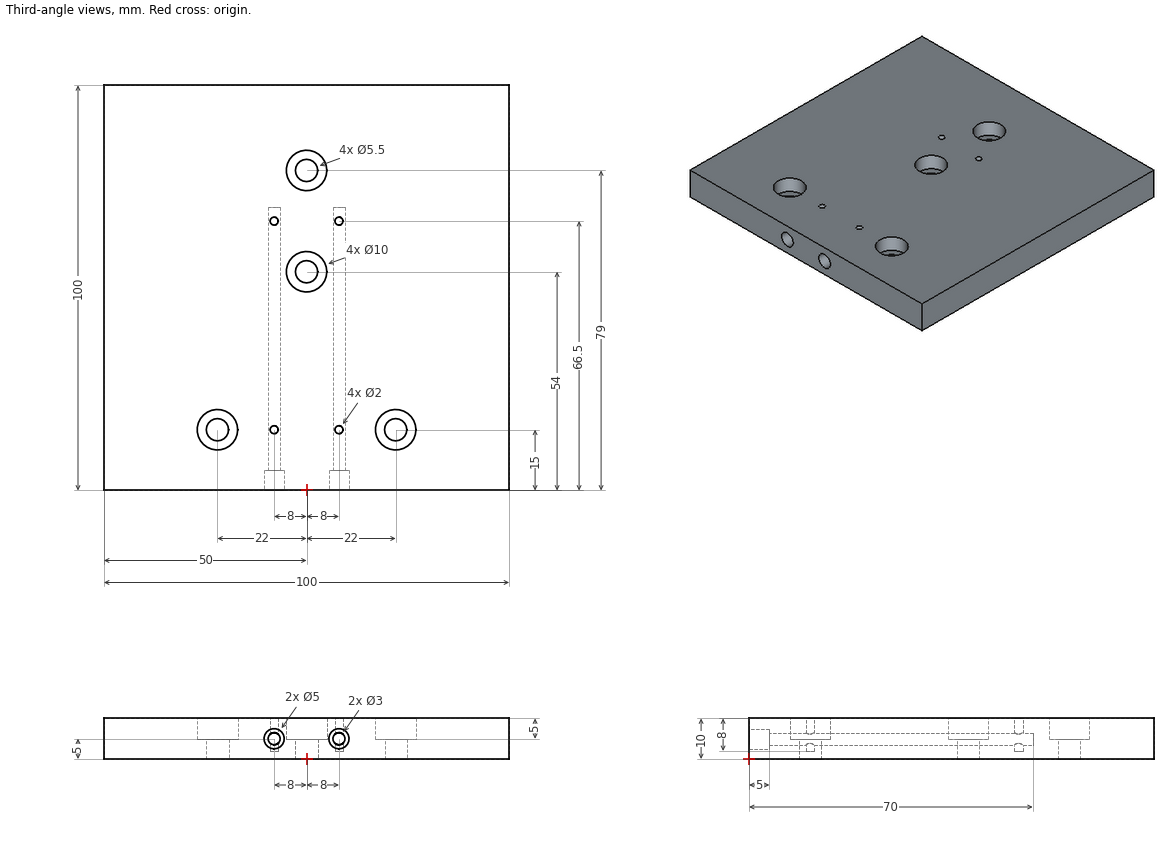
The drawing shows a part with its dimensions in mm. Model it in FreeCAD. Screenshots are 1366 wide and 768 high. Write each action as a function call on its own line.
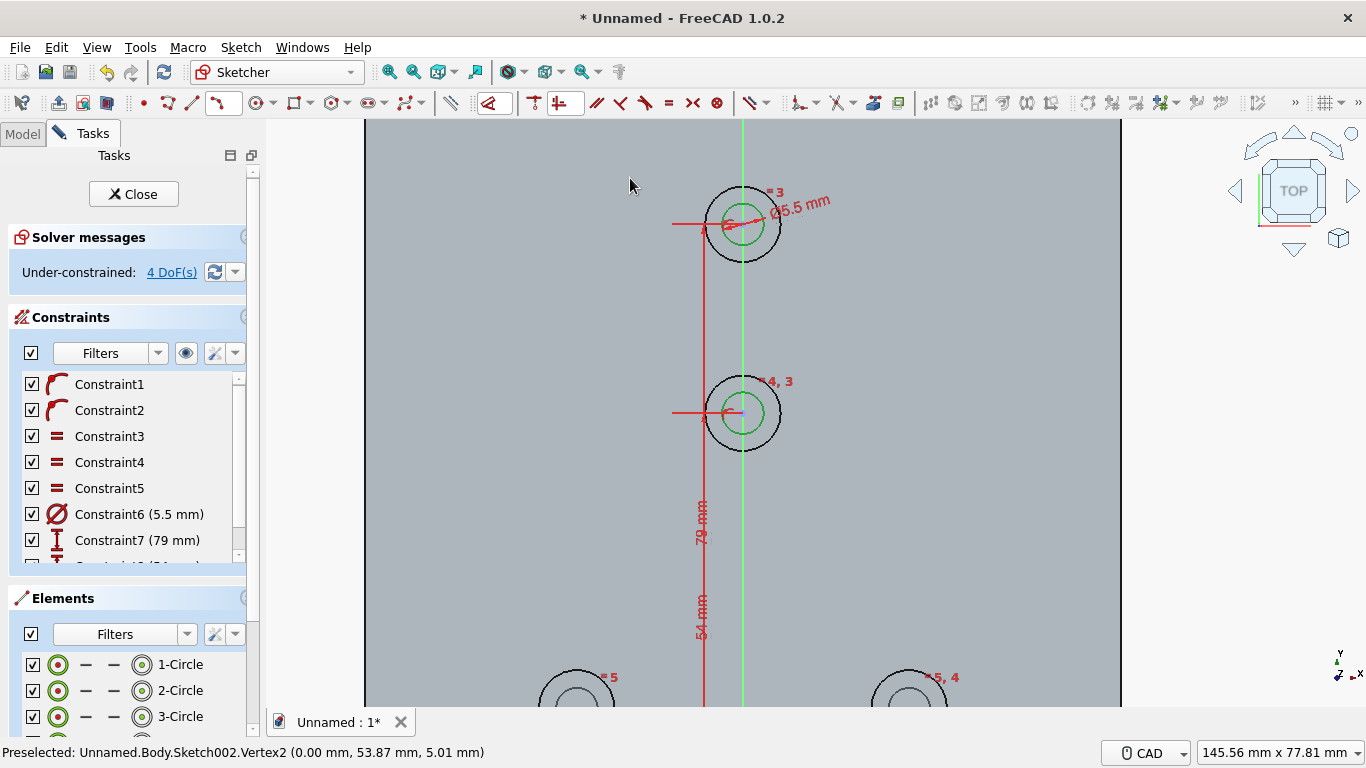
scroll(757, 211, down, 2)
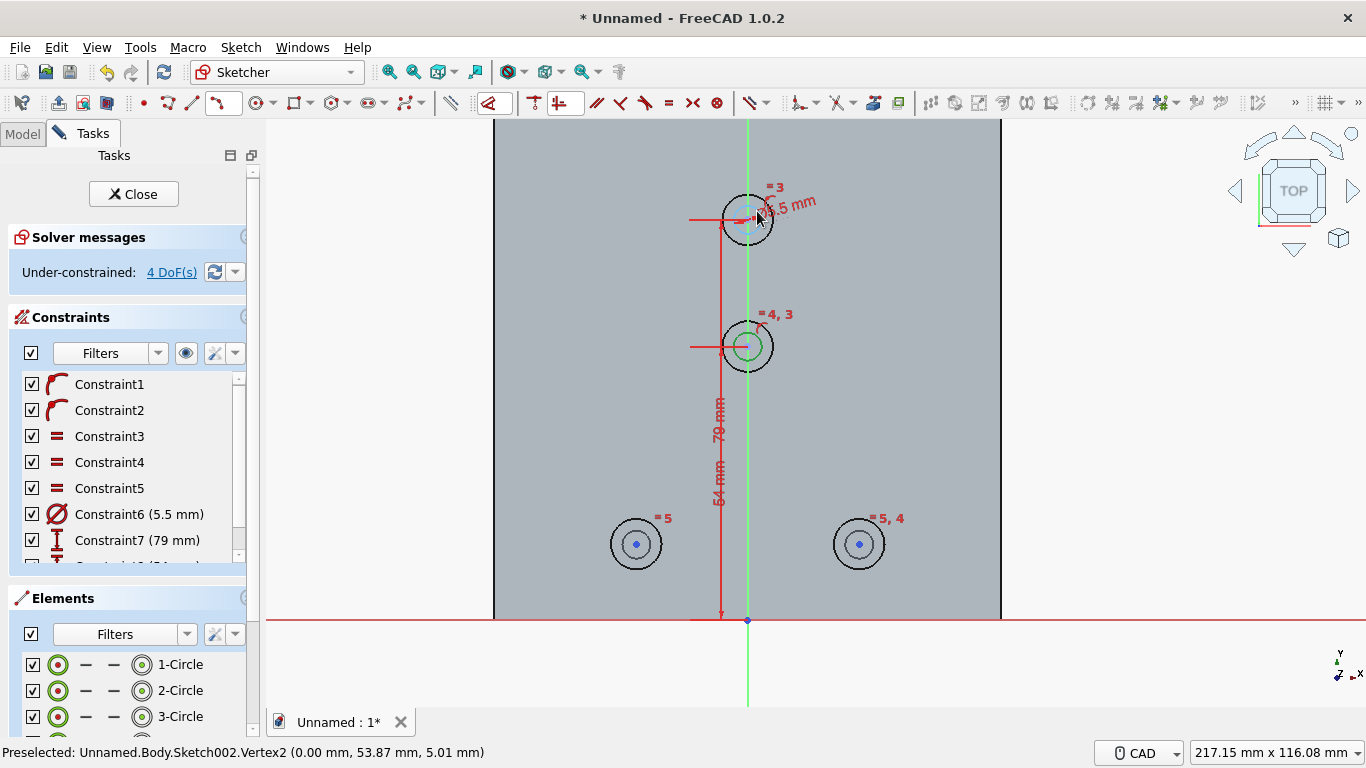
click(859, 545)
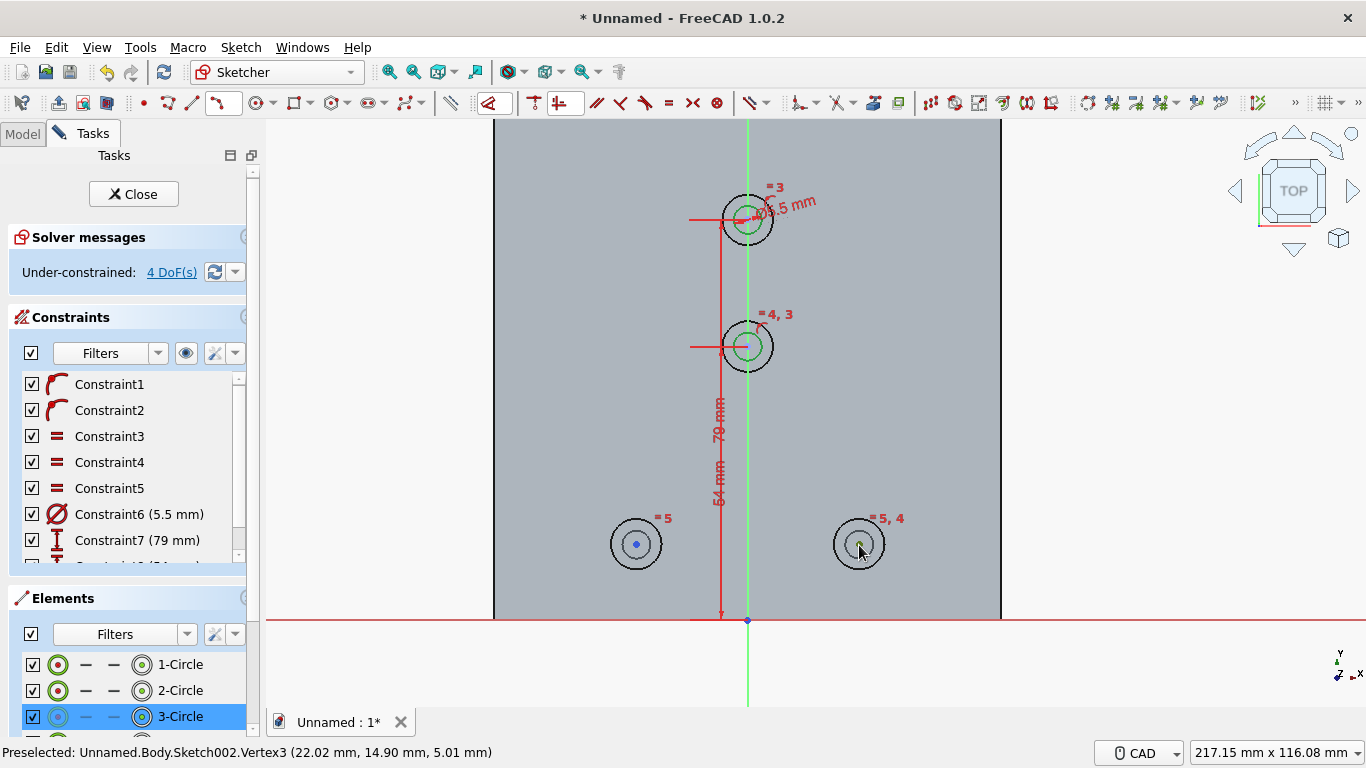
click(506, 104)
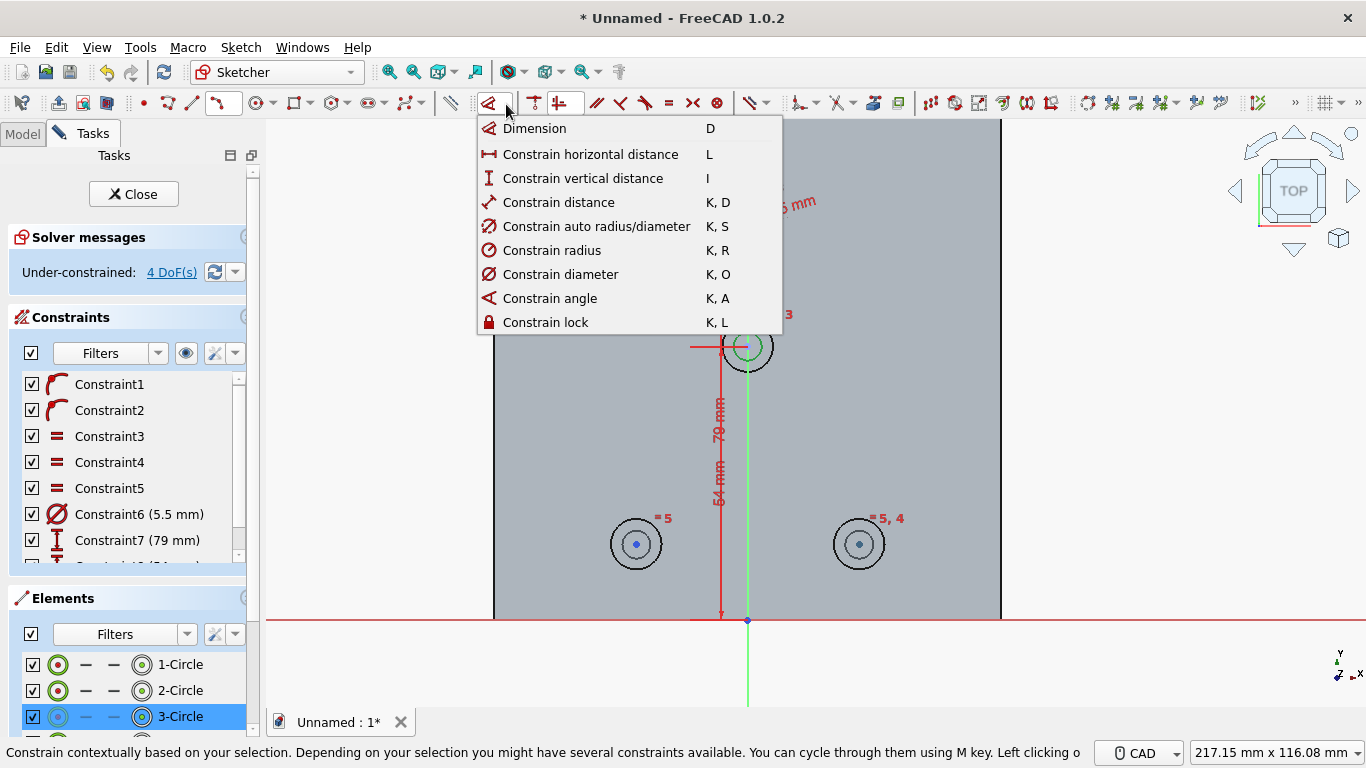
click(630, 154)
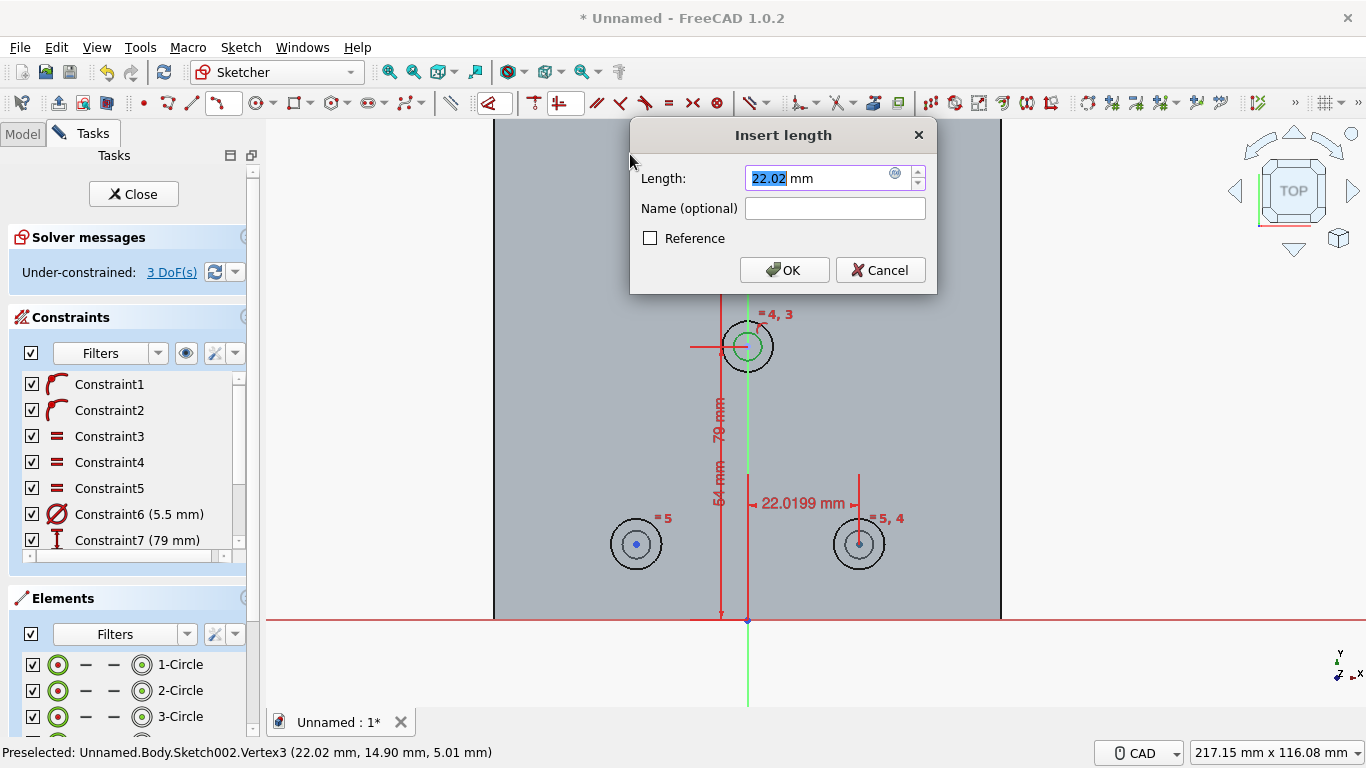
text(22)
key(Return)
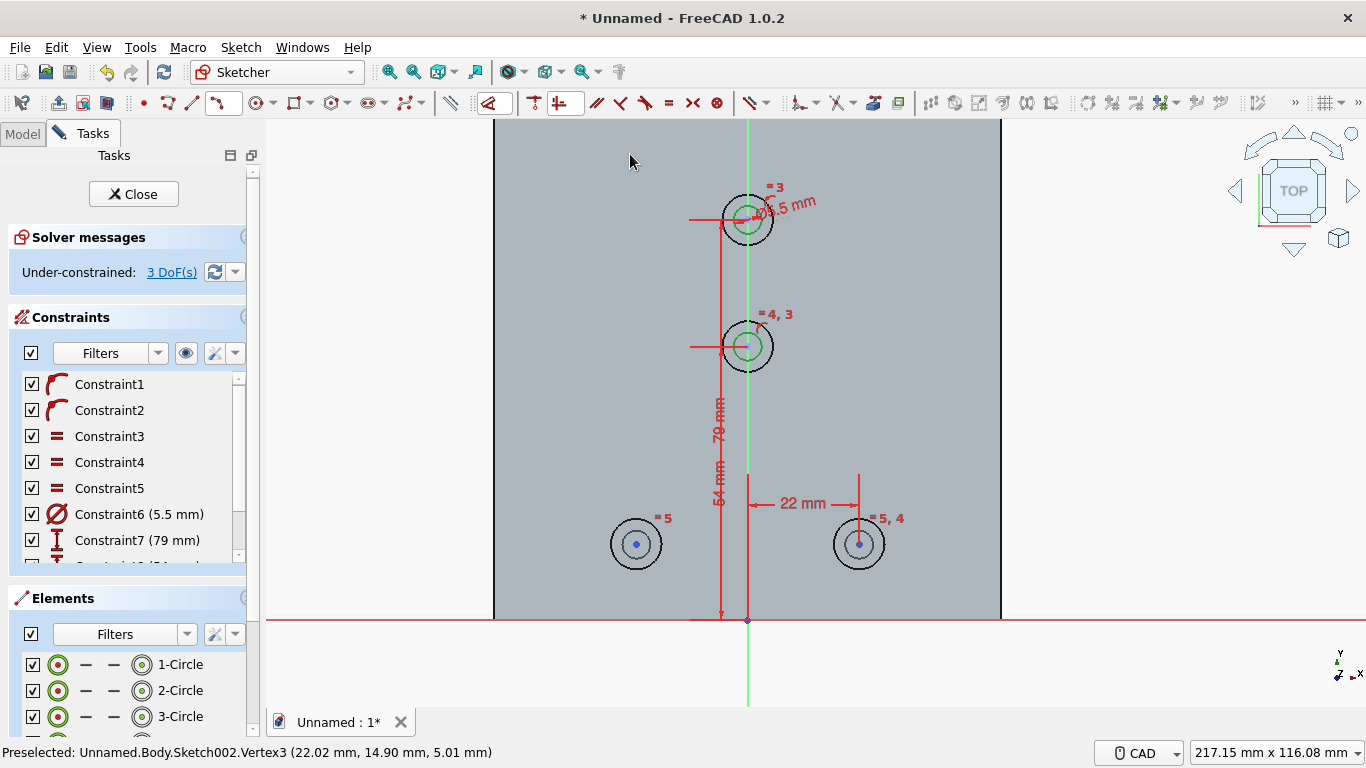
click(859, 545)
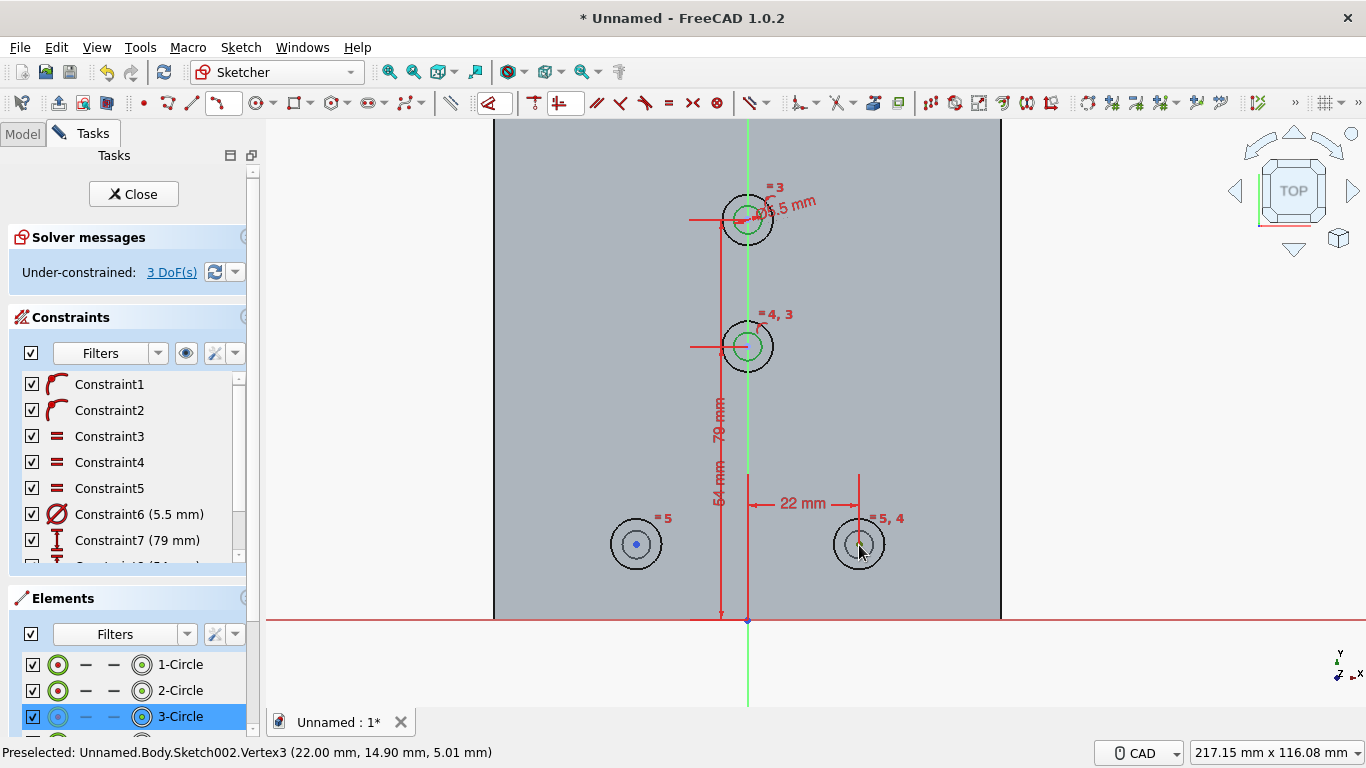
click(506, 104)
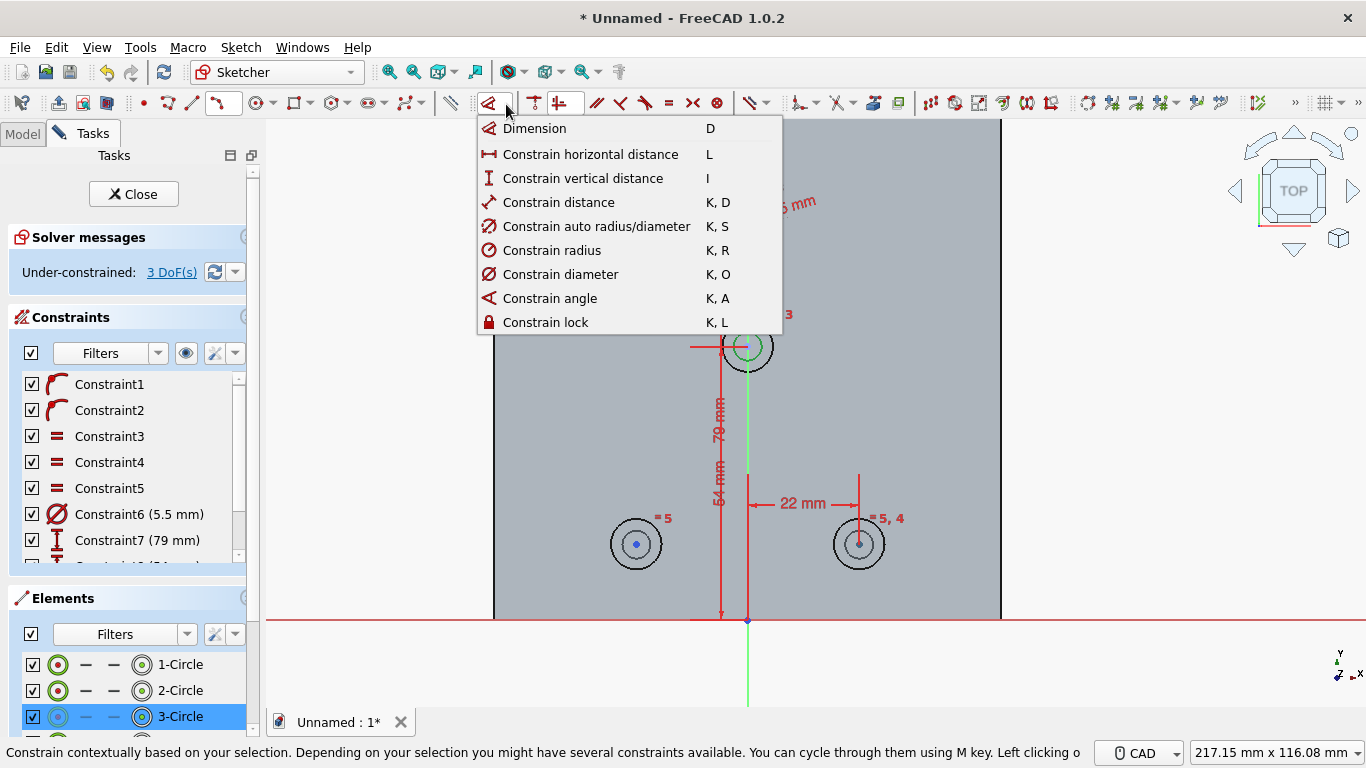
click(630, 178)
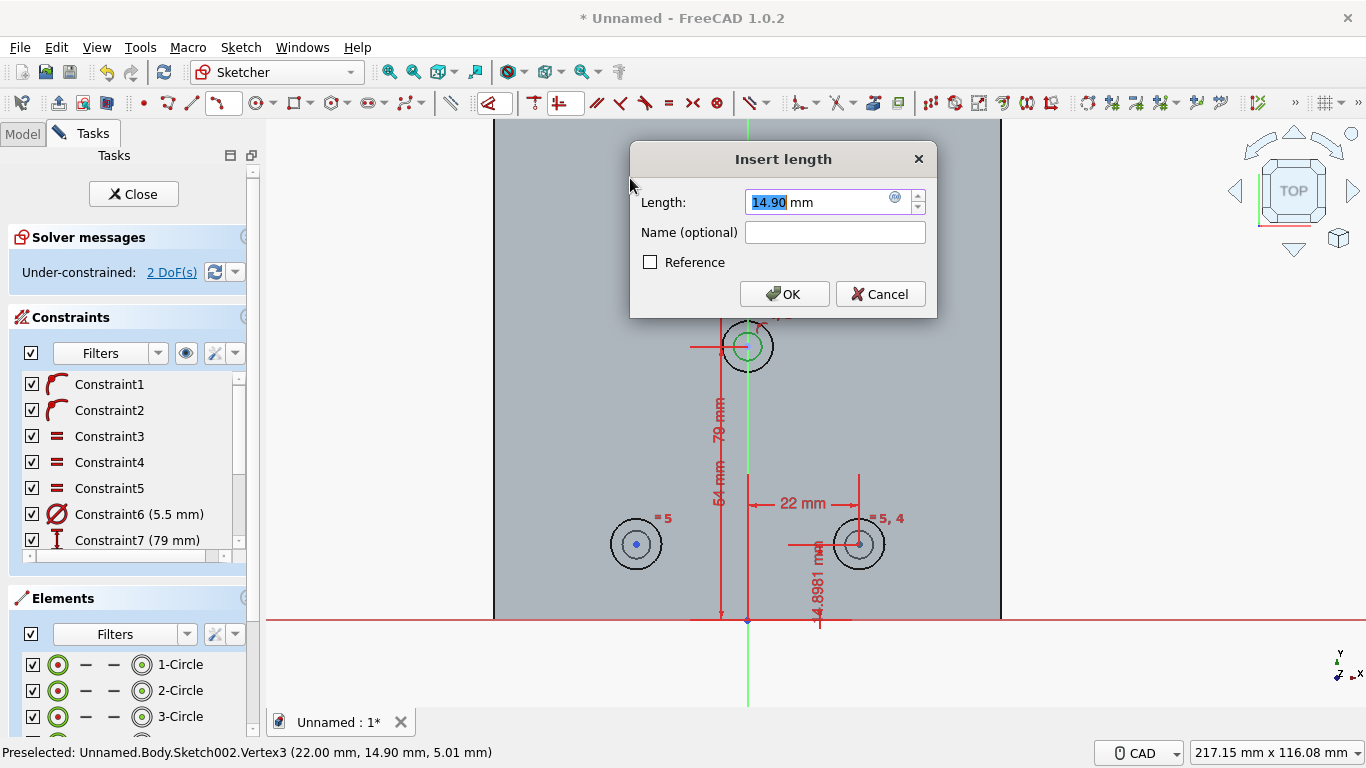
text(15)
key(Return)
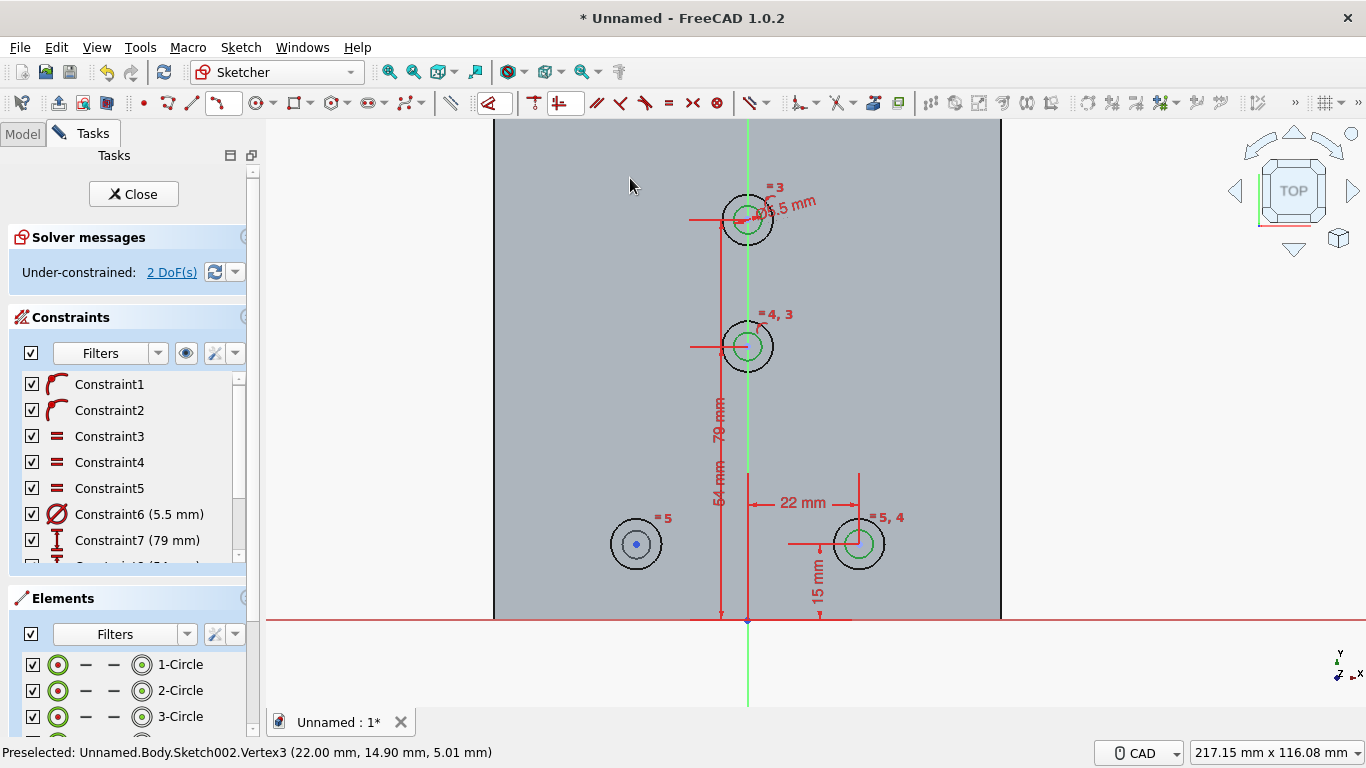
click(636, 545)